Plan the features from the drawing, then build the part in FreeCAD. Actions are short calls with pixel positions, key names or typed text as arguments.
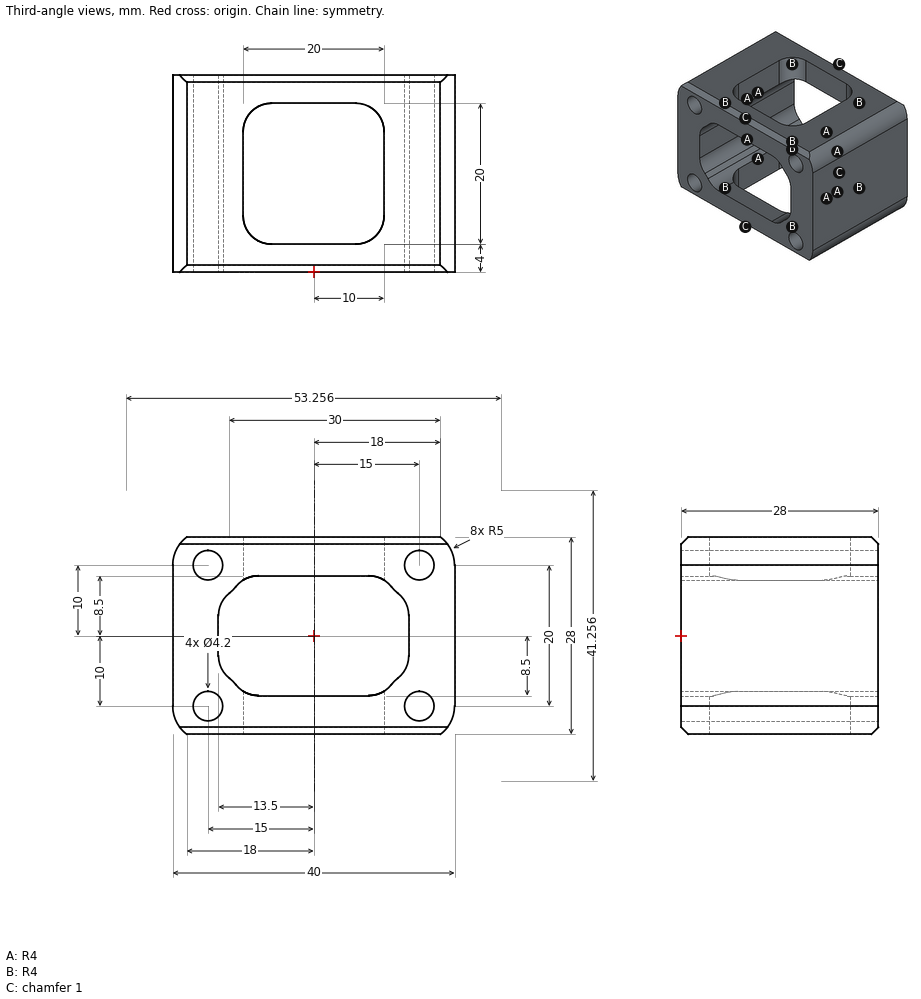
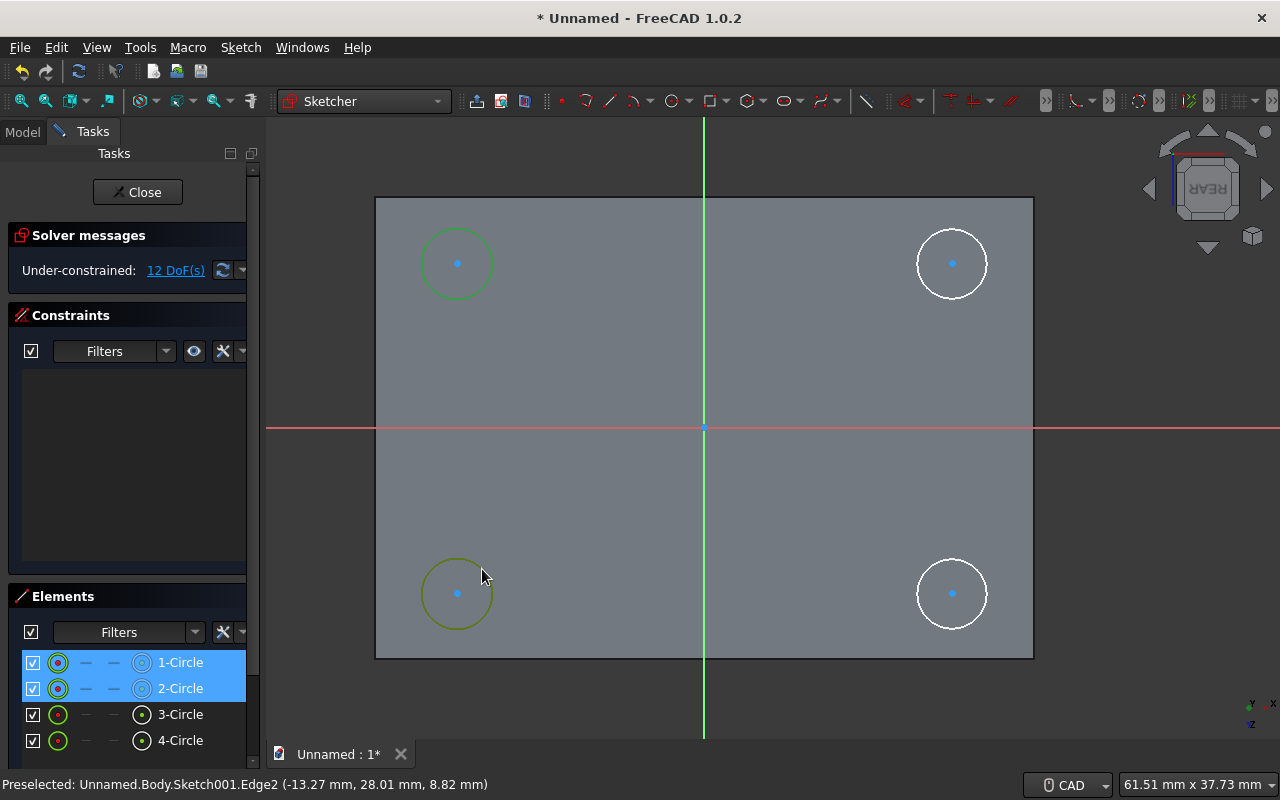
click(976, 569)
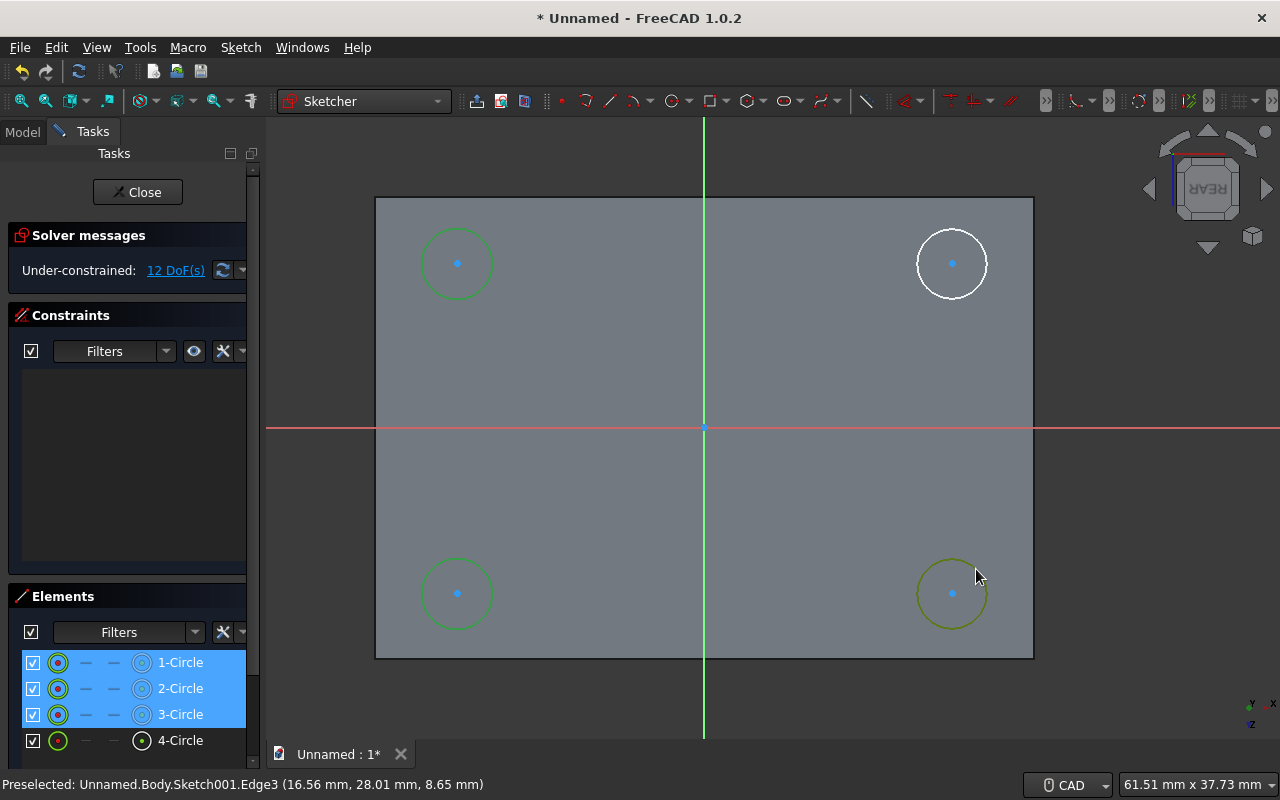
click(976, 239)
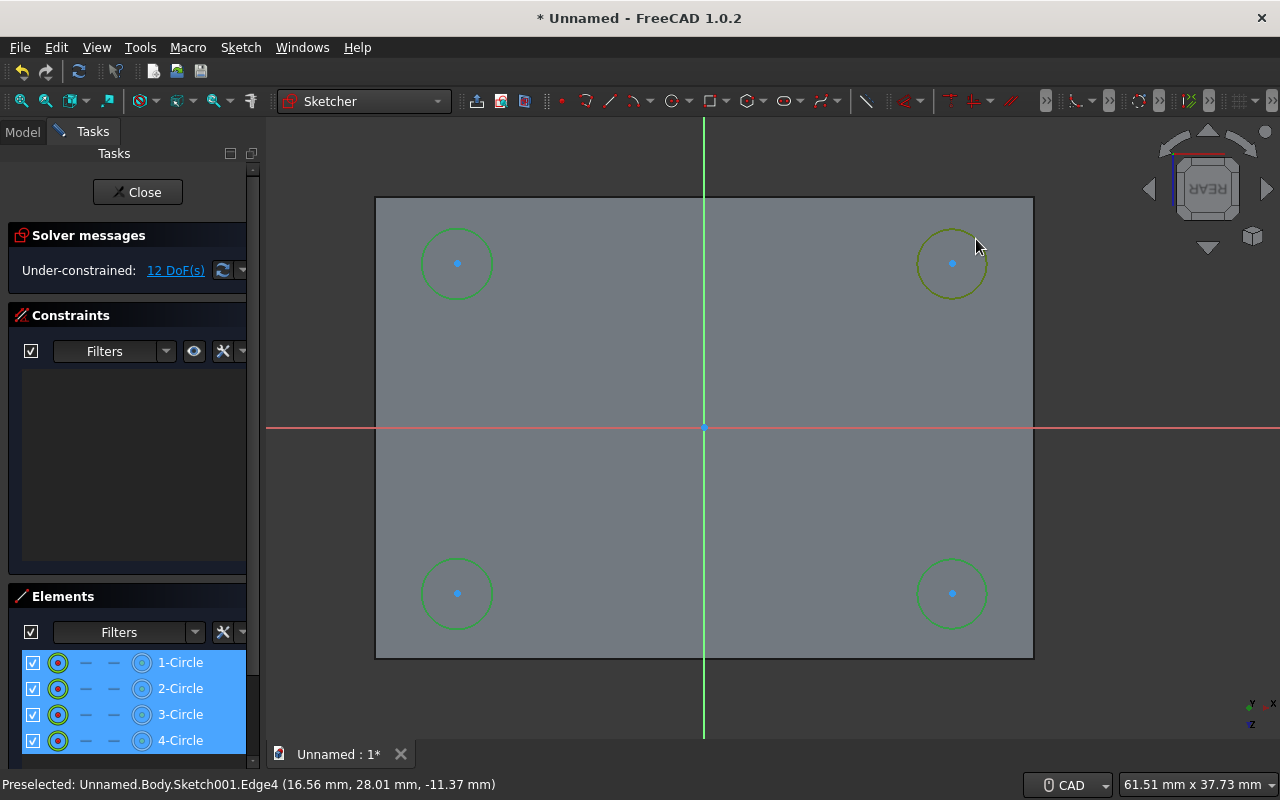
key(e)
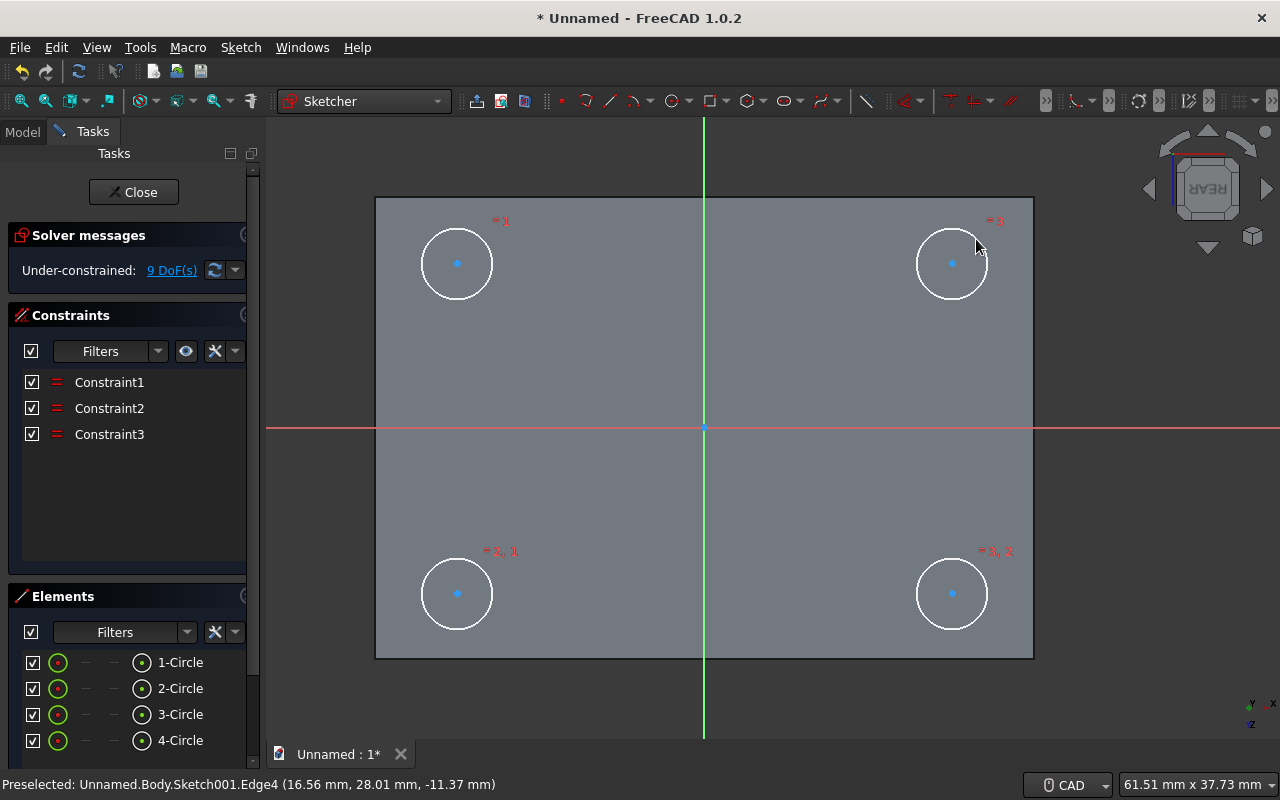
click(457, 264)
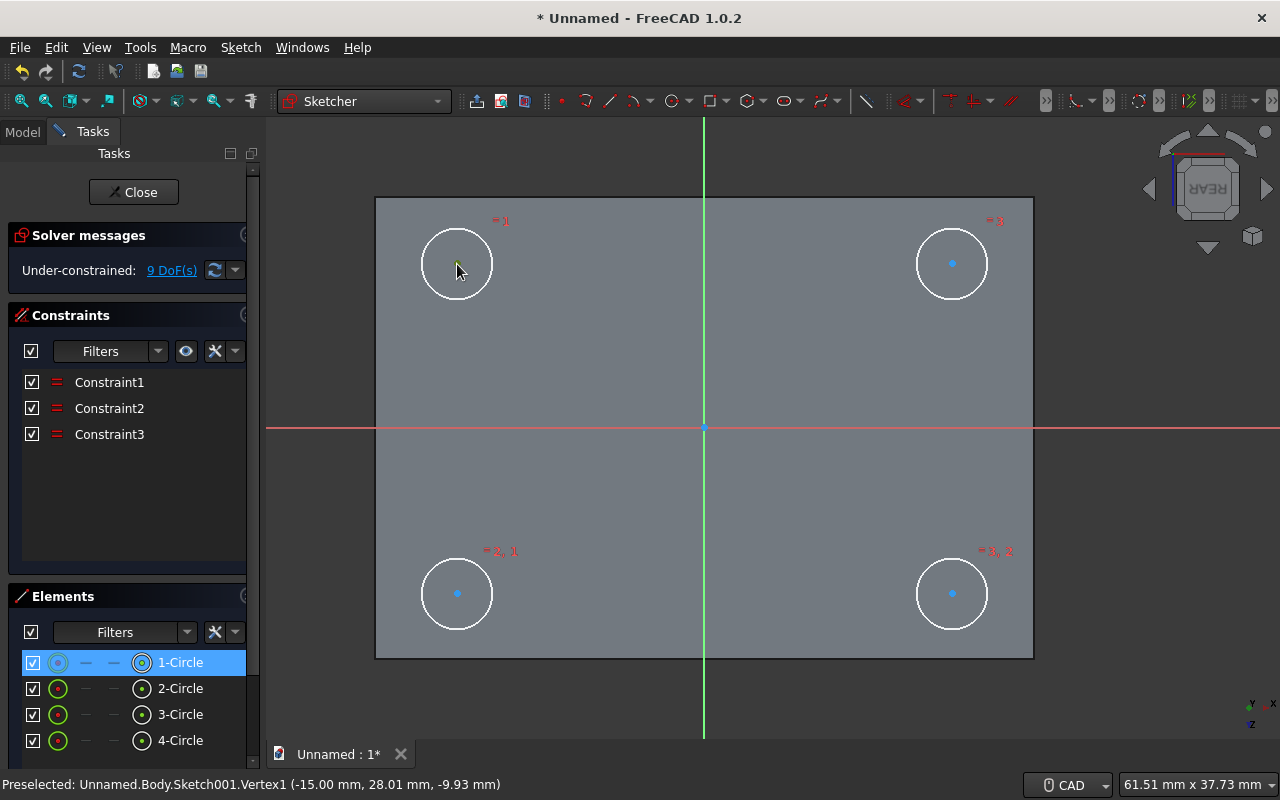
click(457, 594)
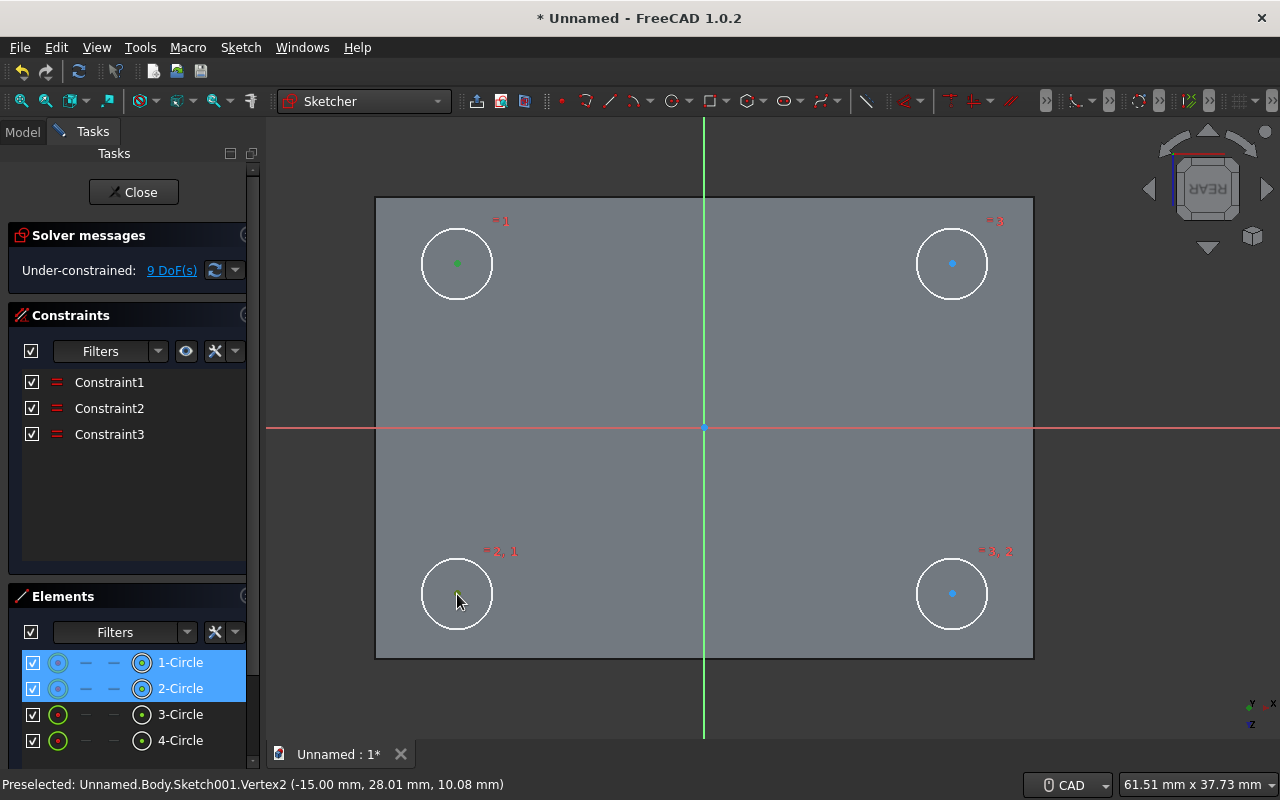
key(v)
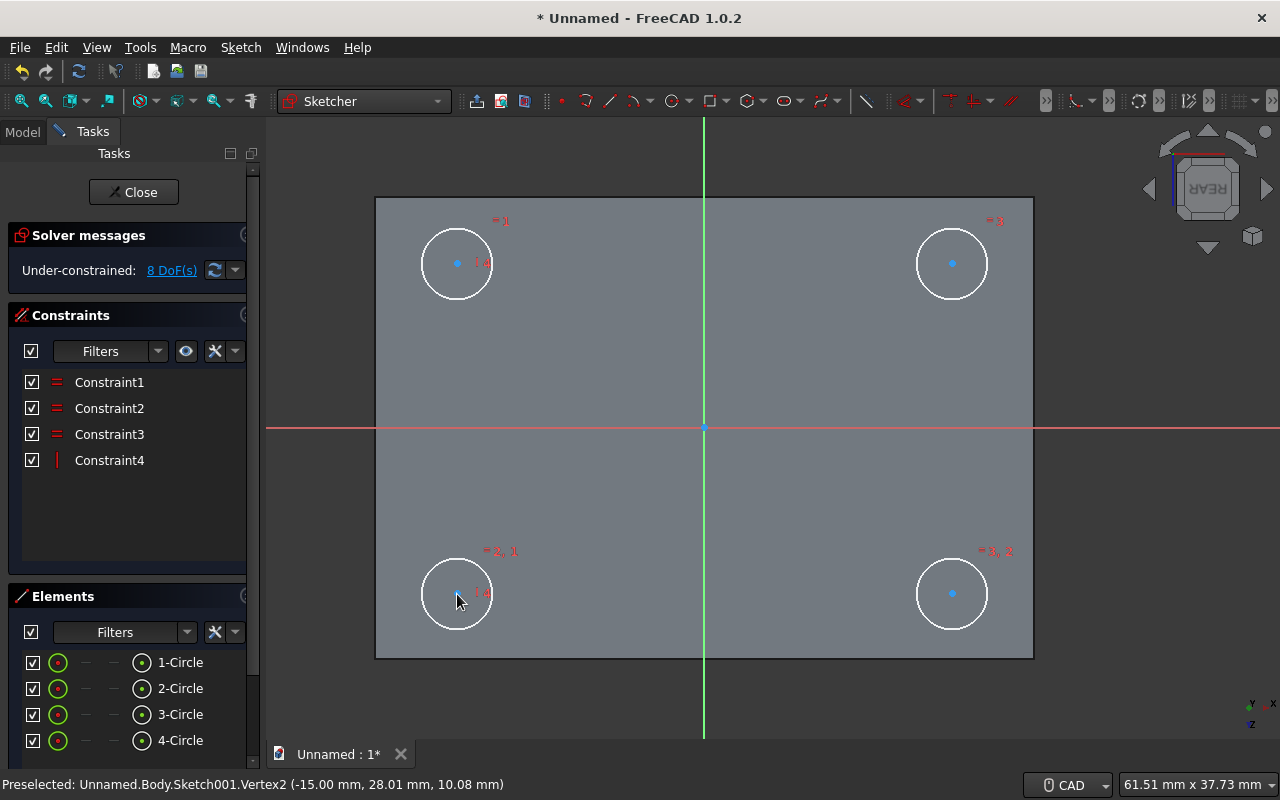
click(457, 594)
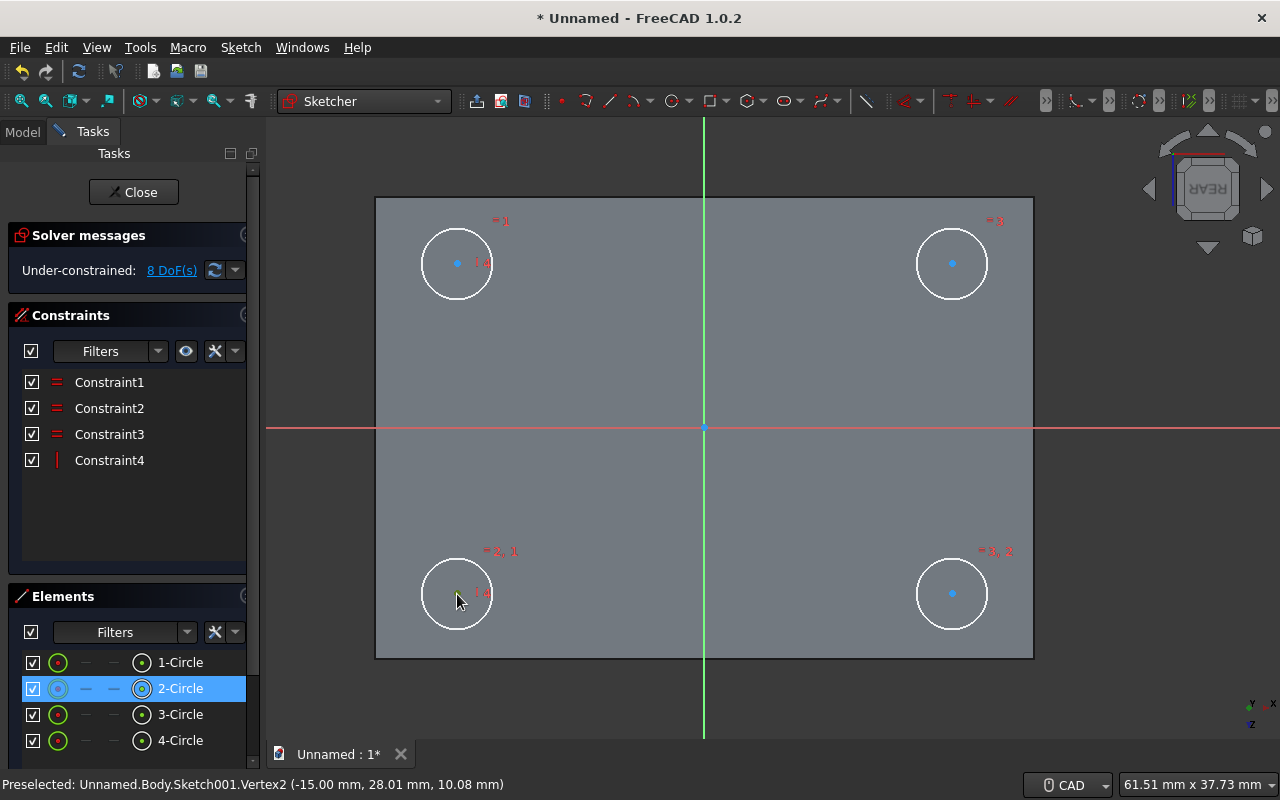
click(952, 594)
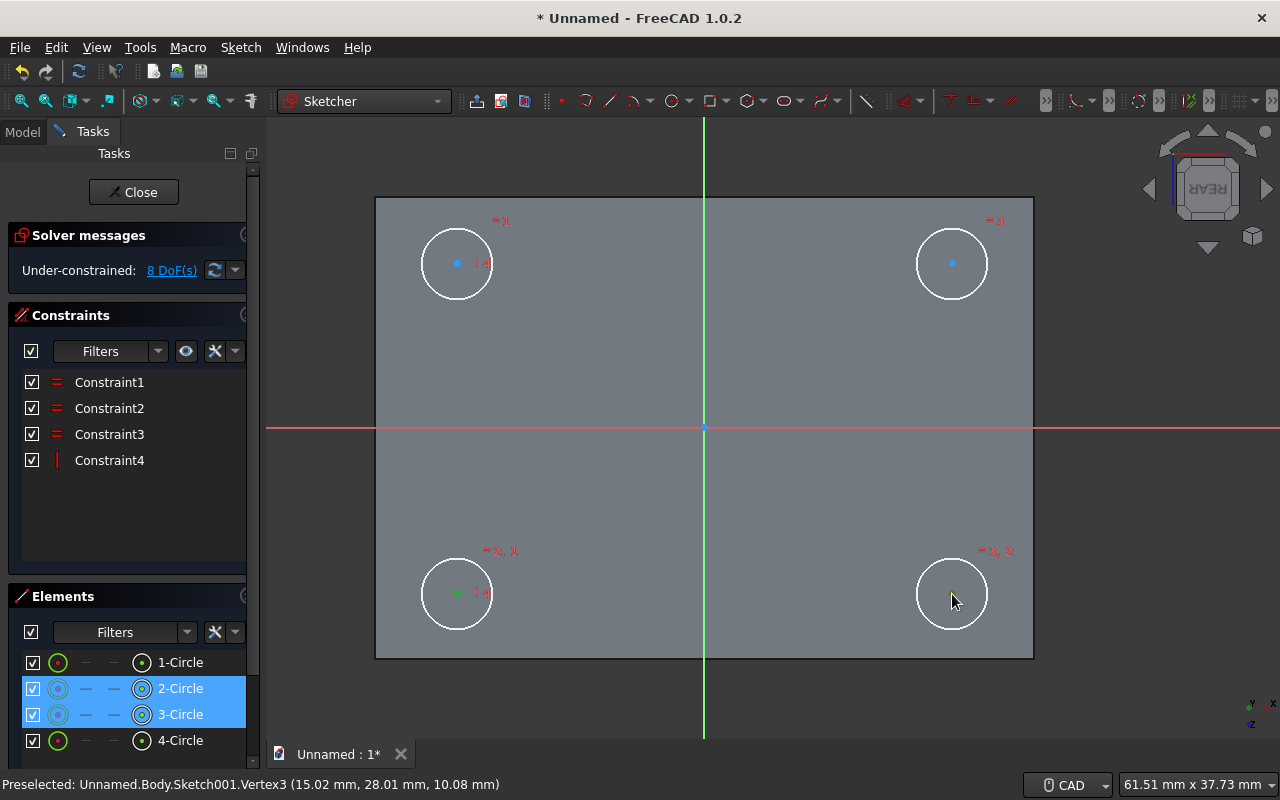
key(h)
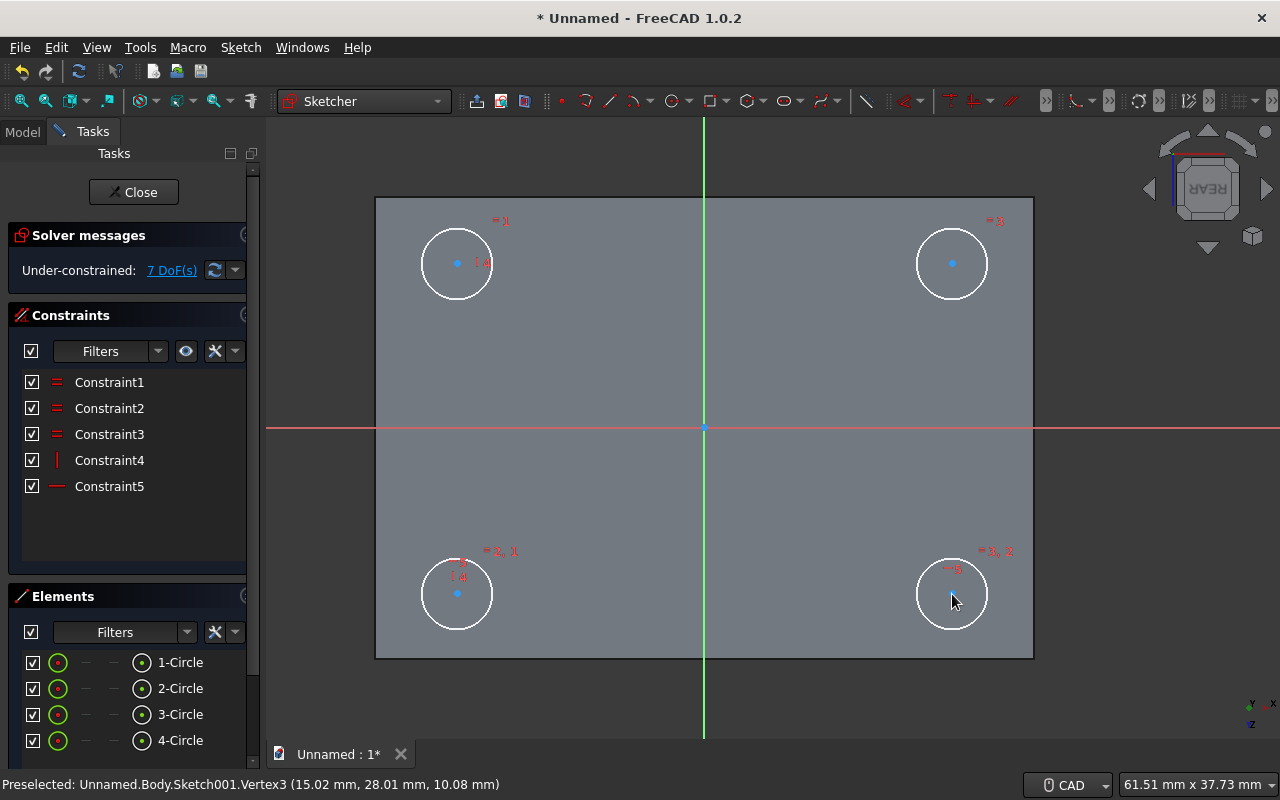
click(952, 594)